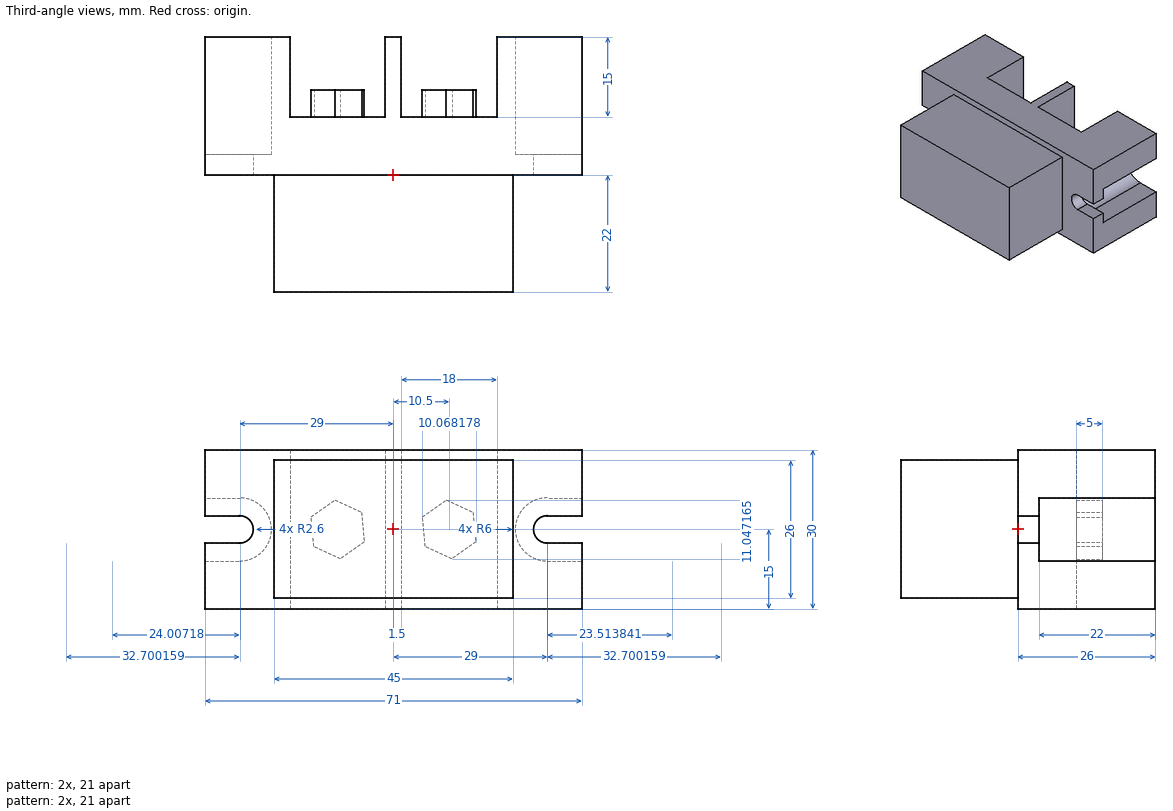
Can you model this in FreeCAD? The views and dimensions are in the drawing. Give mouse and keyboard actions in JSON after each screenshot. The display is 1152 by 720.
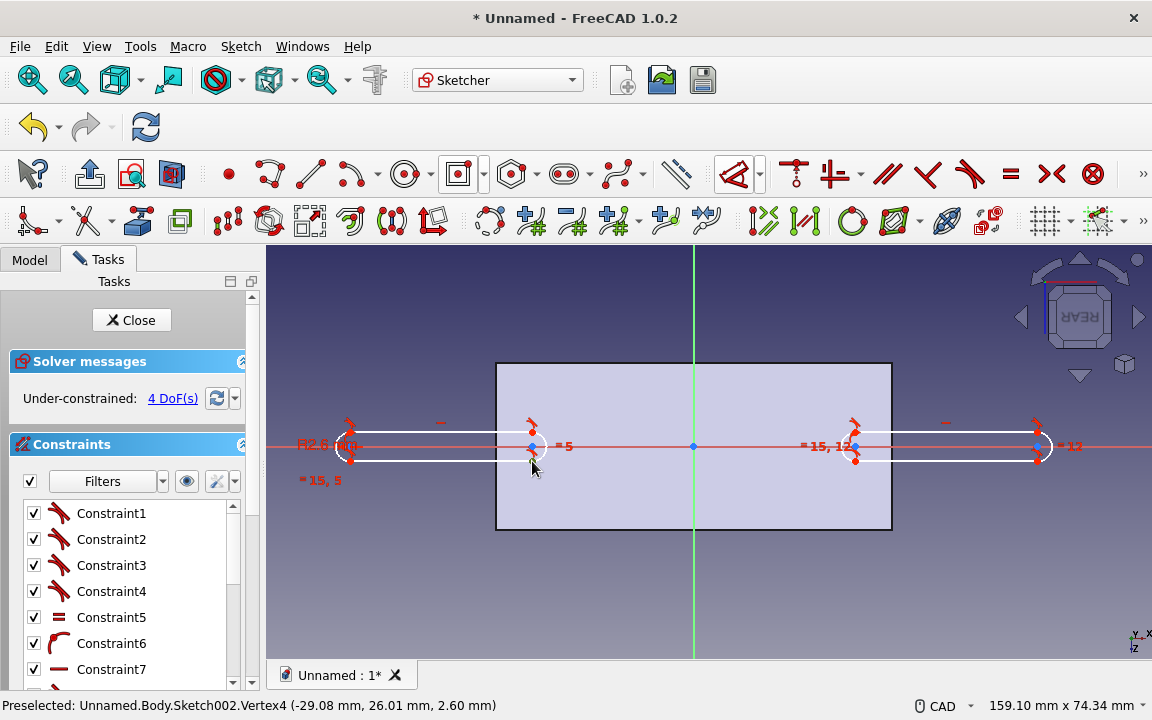
{"action": "left_click", "coordinate": [760, 174]}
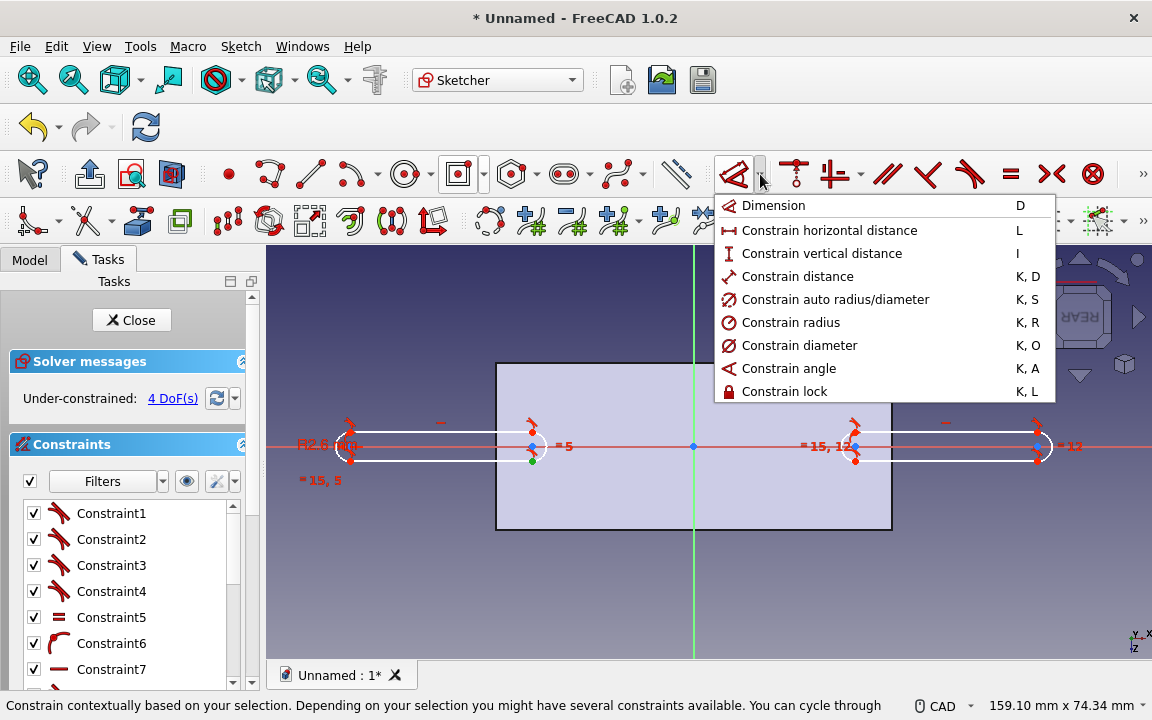
{"action": "left_click", "coordinate": [885, 230]}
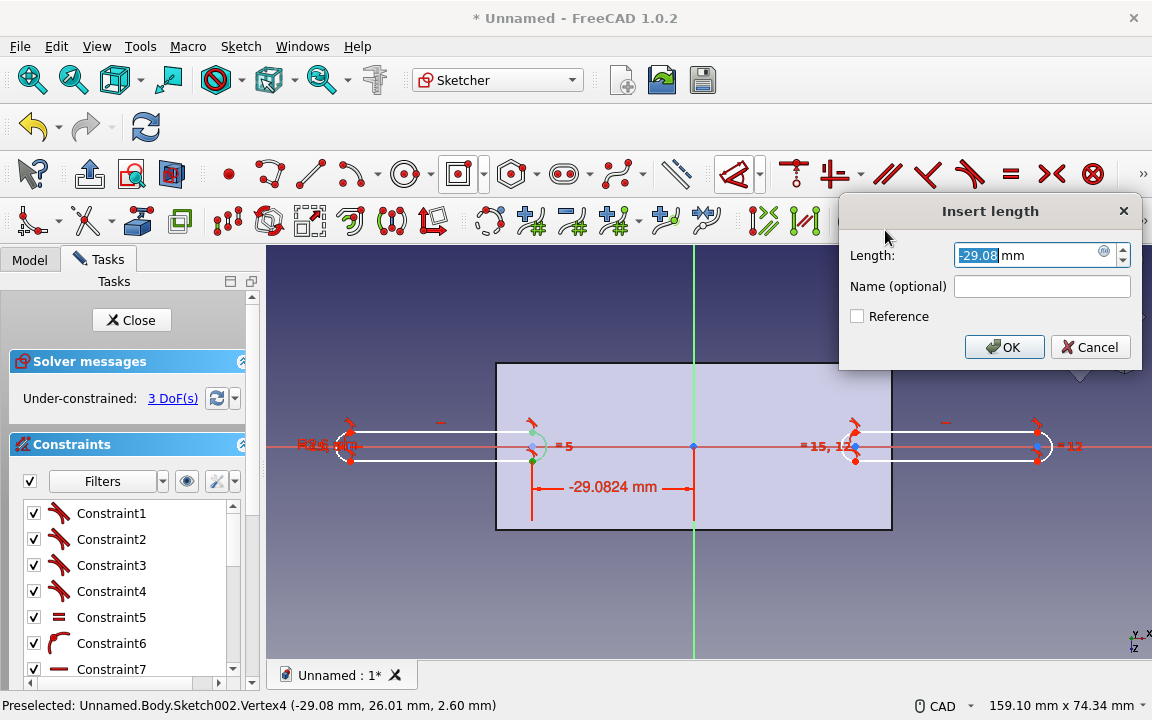
{"action": "type", "text": "-29"}
{"action": "key", "text": "Return"}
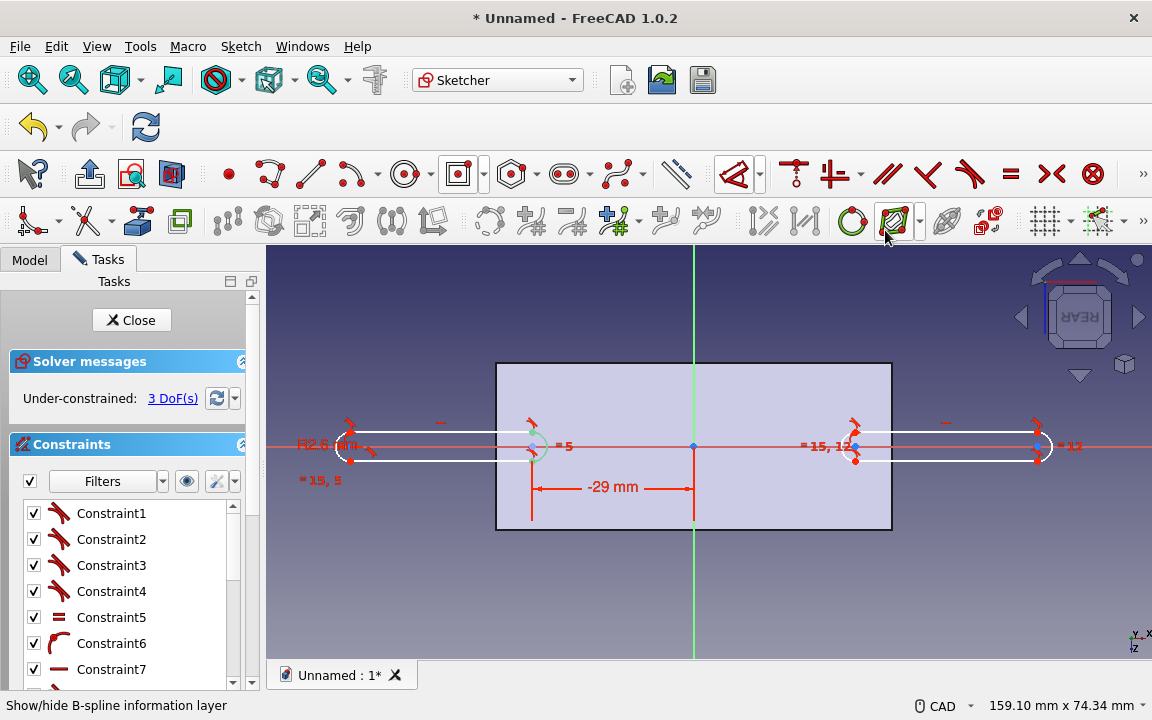
{"action": "left_click", "coordinate": [856, 432]}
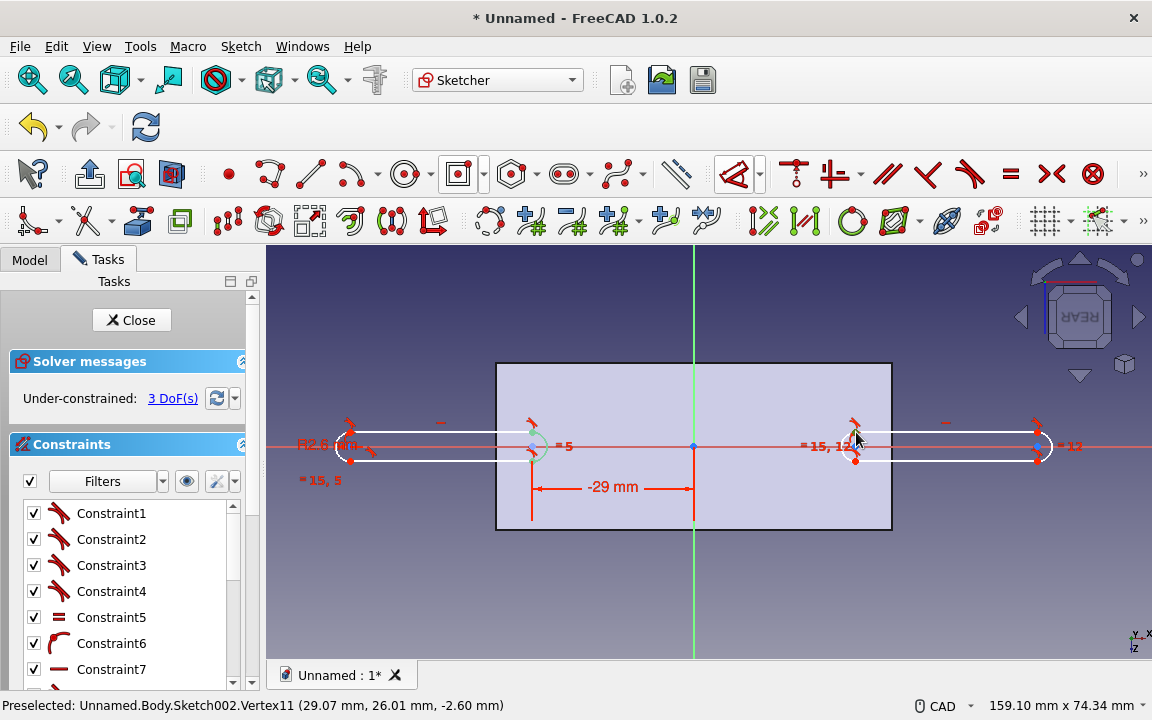
{"action": "key", "text": "l"}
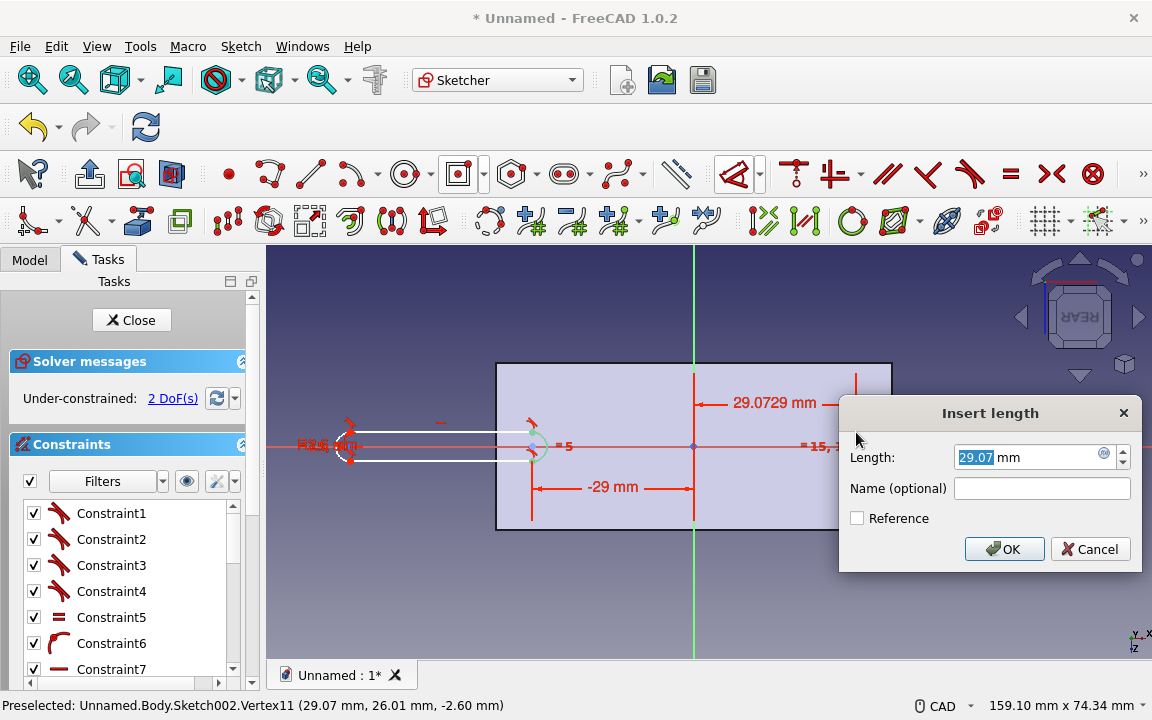
{"action": "type", "text": "29"}
{"action": "key", "text": "Return"}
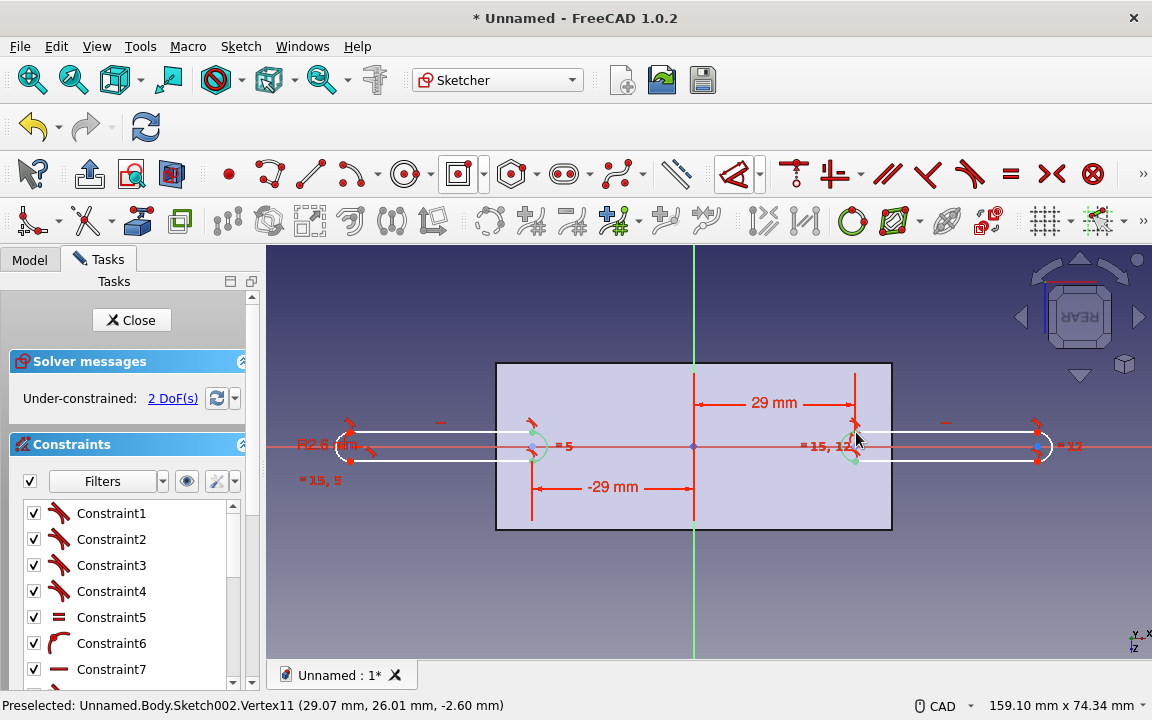
{"action": "left_click", "coordinate": [405, 432]}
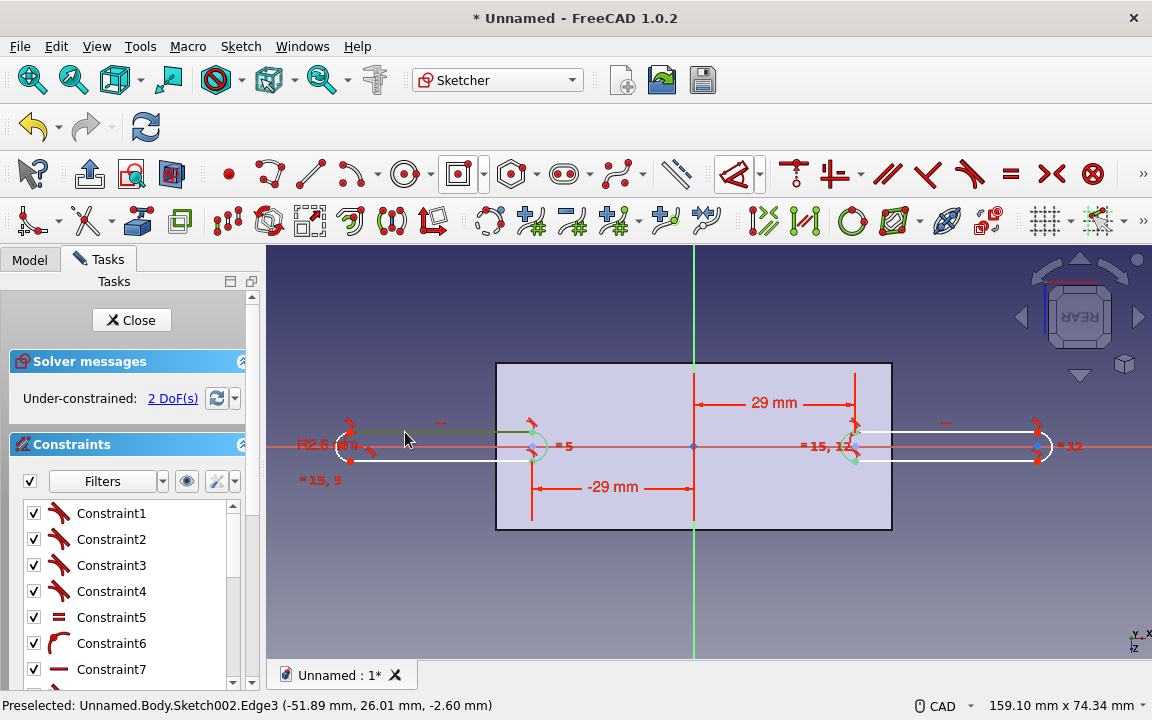
{"action": "key", "text": "l"}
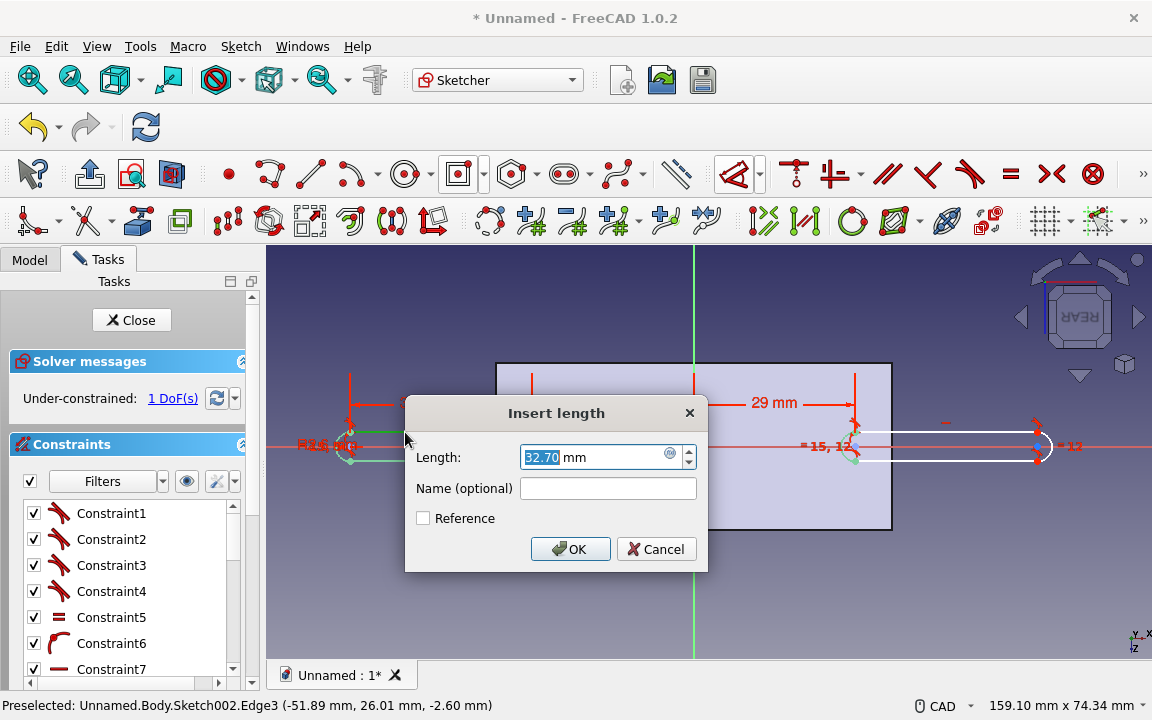
{"action": "type", "text": "32.700159"}
{"action": "key", "text": "Return"}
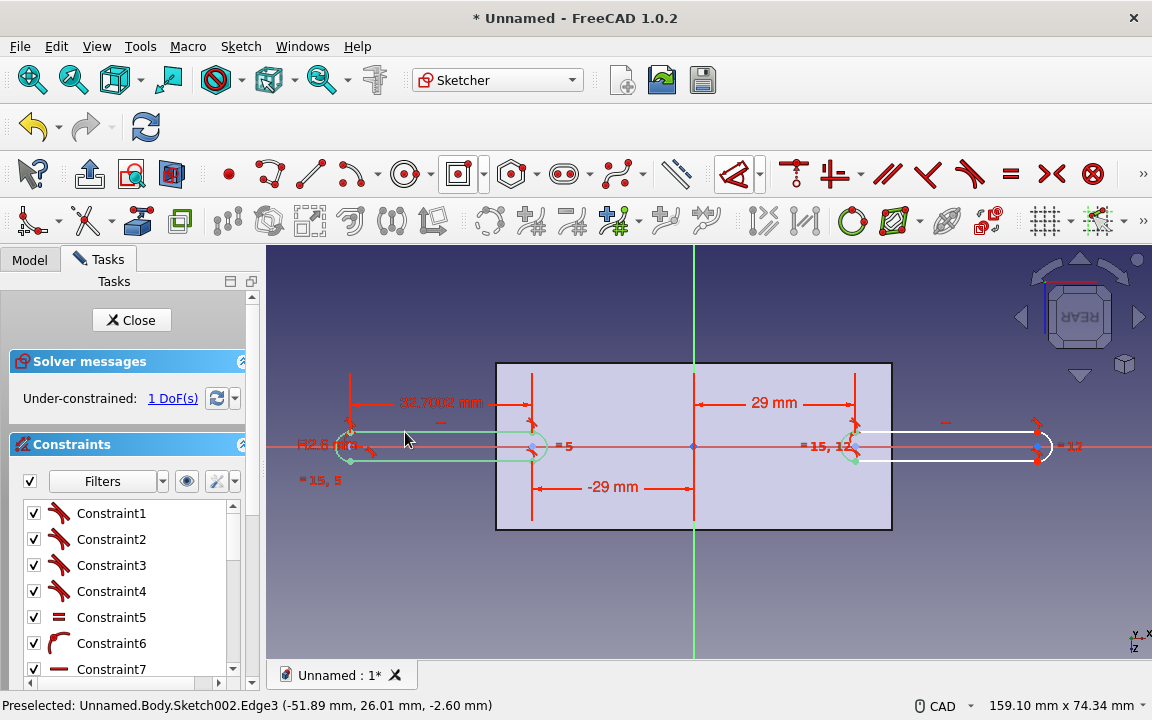
{"action": "left_click", "coordinate": [910, 432]}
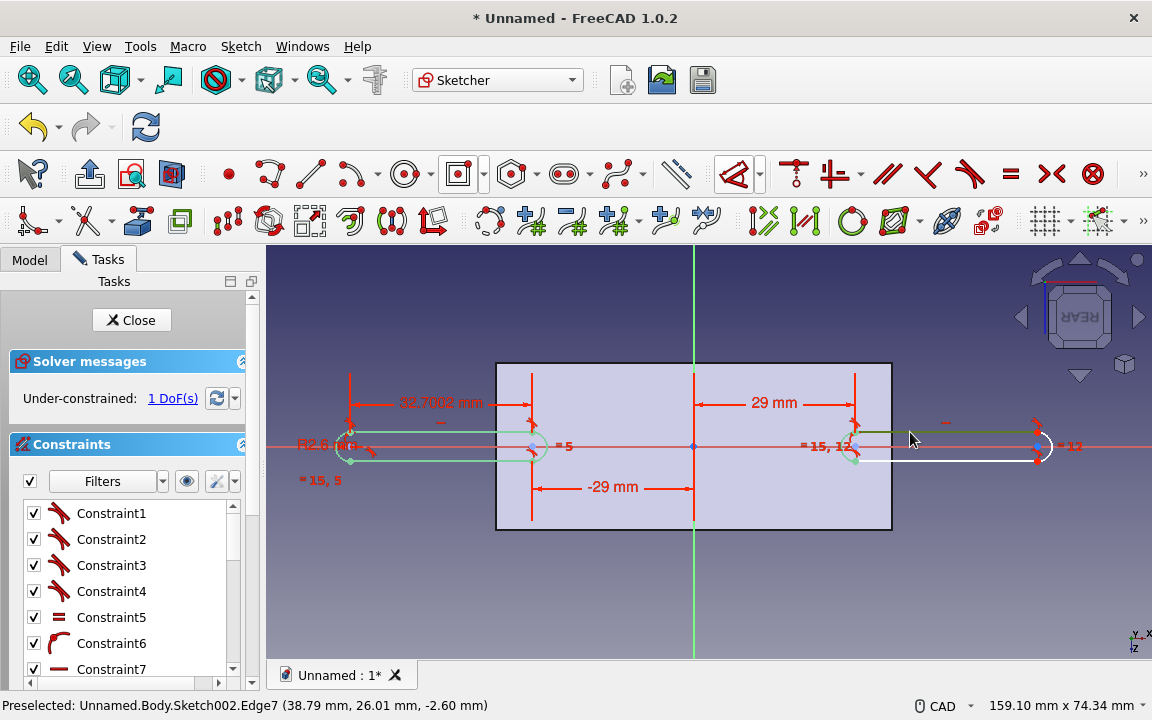
{"action": "key", "text": "l"}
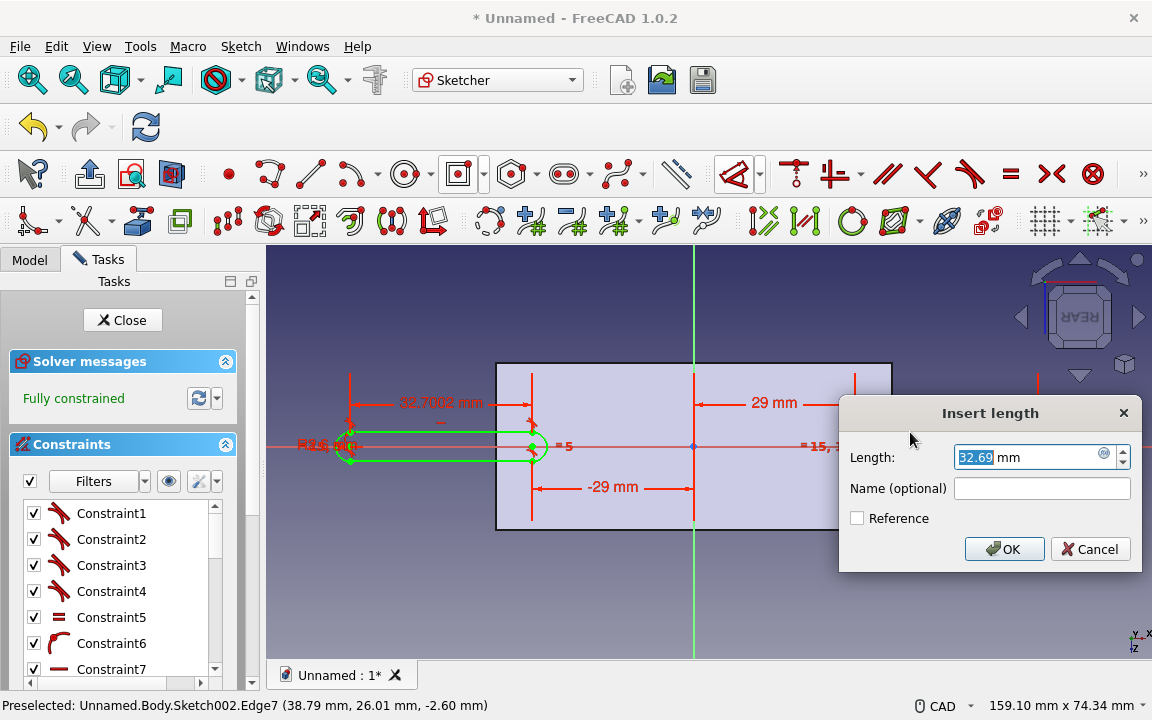
{"action": "type", "text": "32.700159"}
{"action": "key", "text": "Return"}